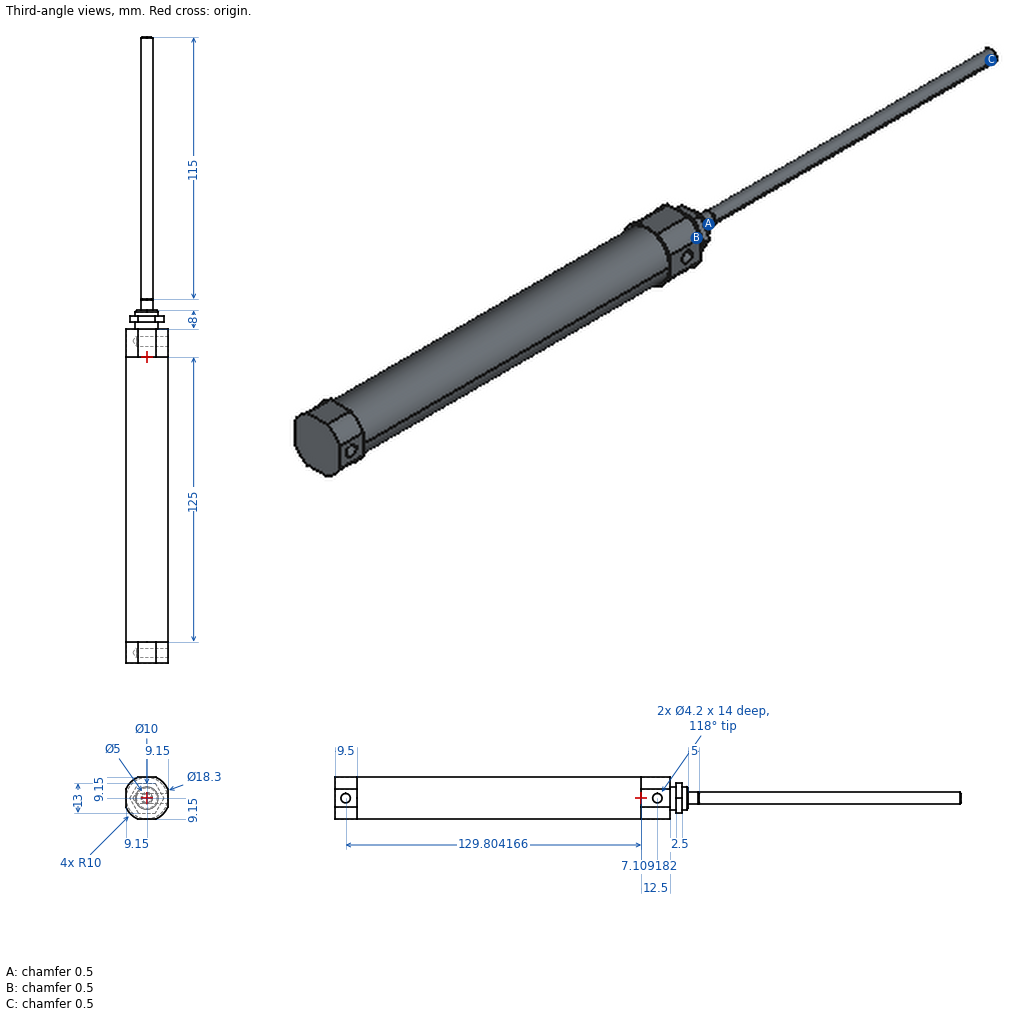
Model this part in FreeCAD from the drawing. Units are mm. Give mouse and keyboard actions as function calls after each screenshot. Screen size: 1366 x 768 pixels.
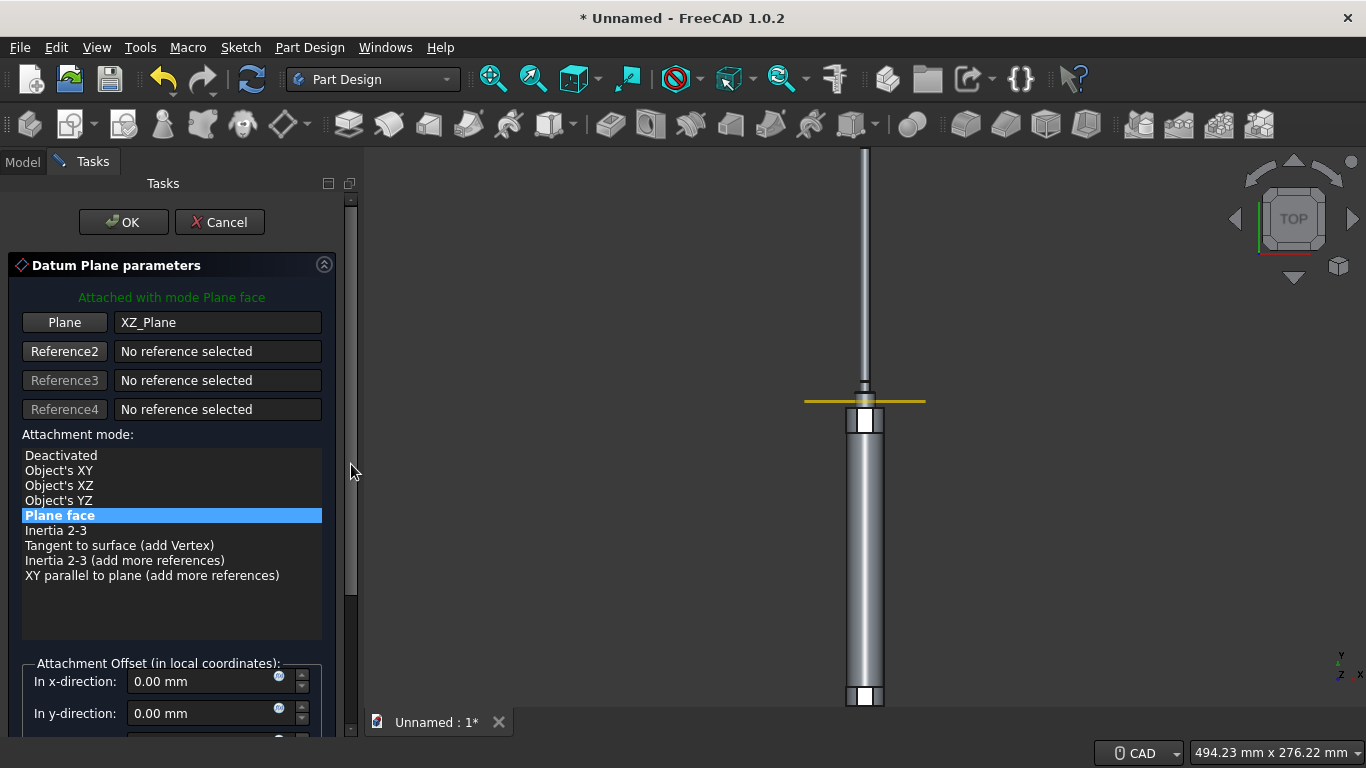
click(124, 222)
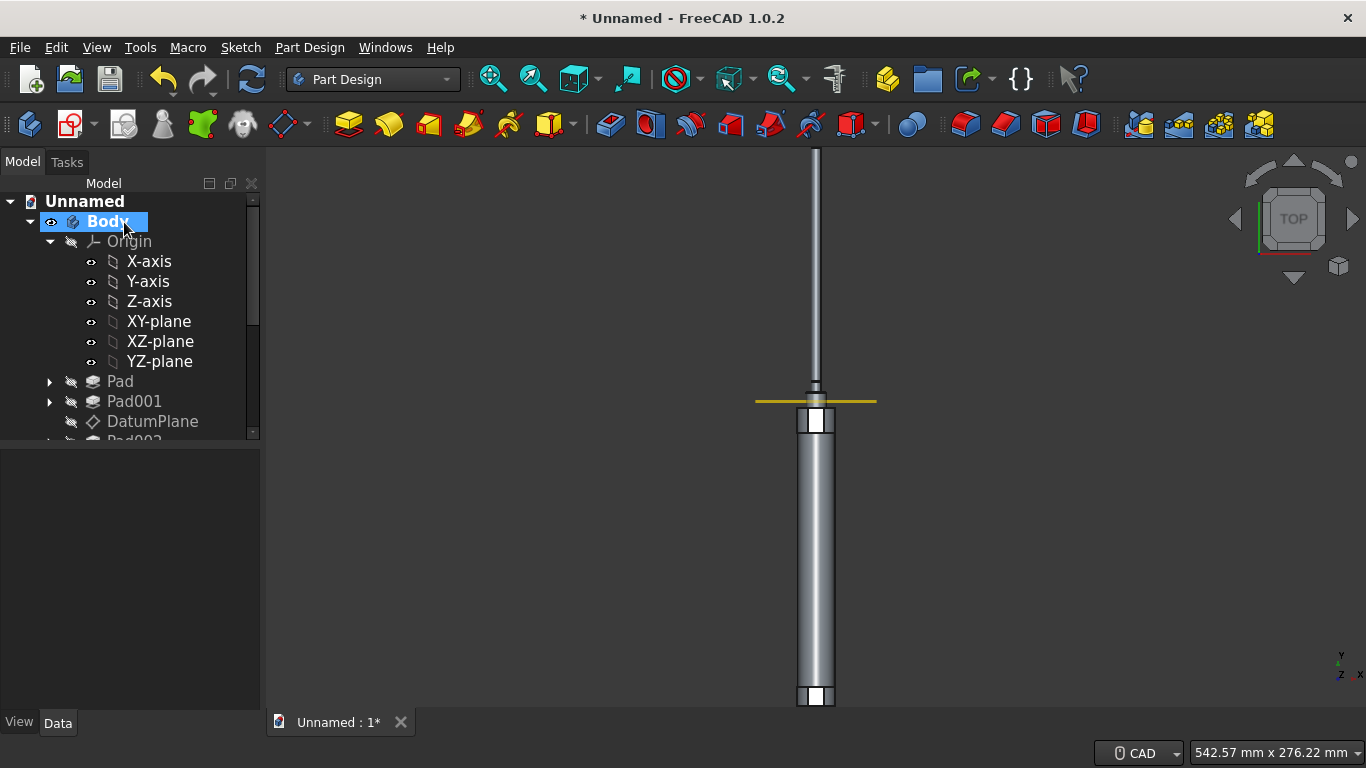
scroll(100, 317, down, 3)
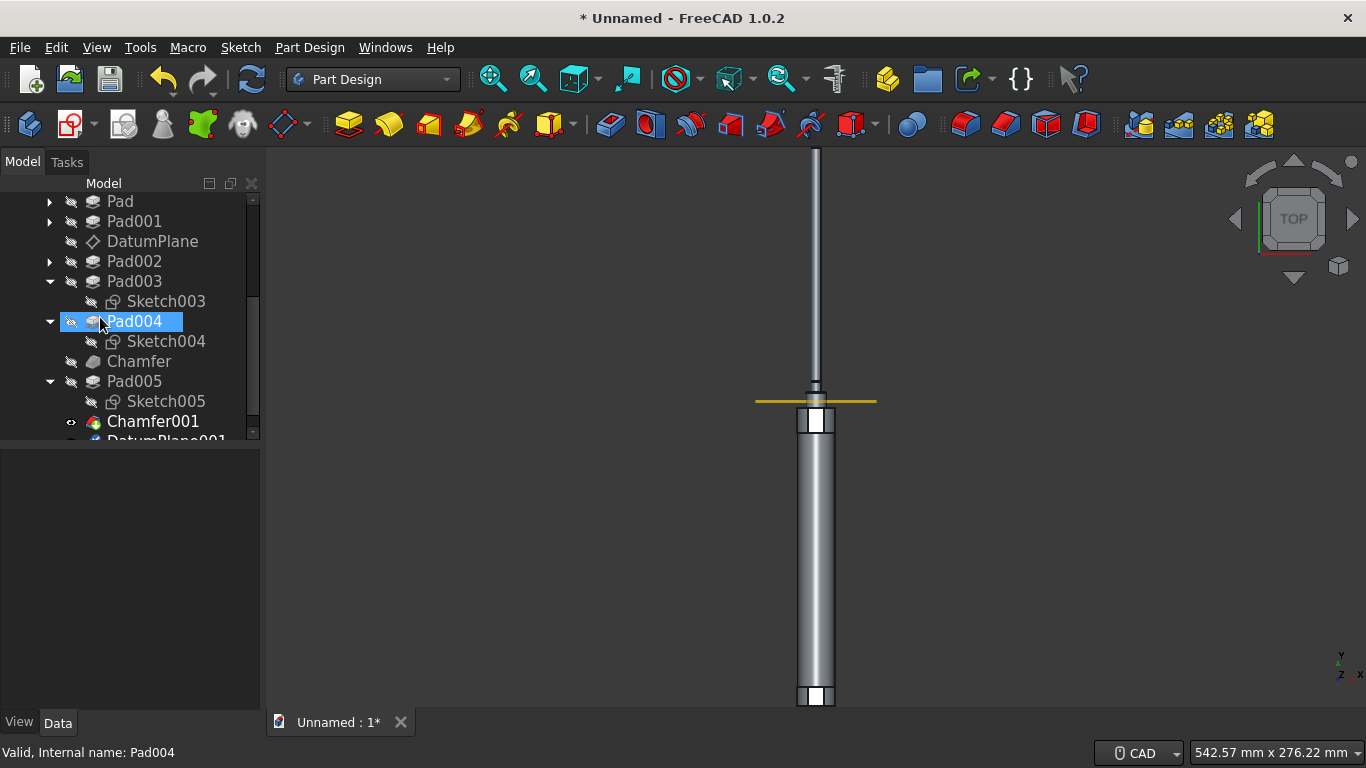
scroll(140, 317, up, 15)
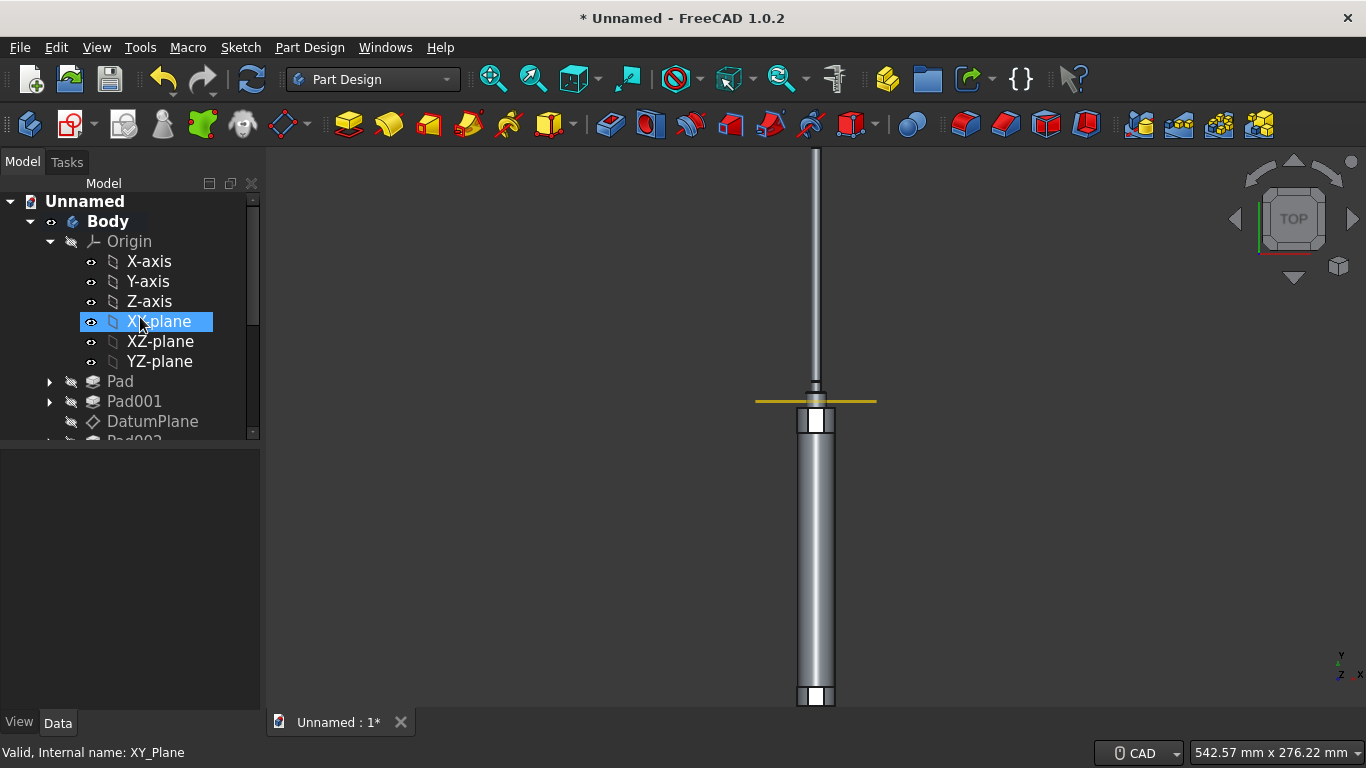
scroll(100, 317, down, 6)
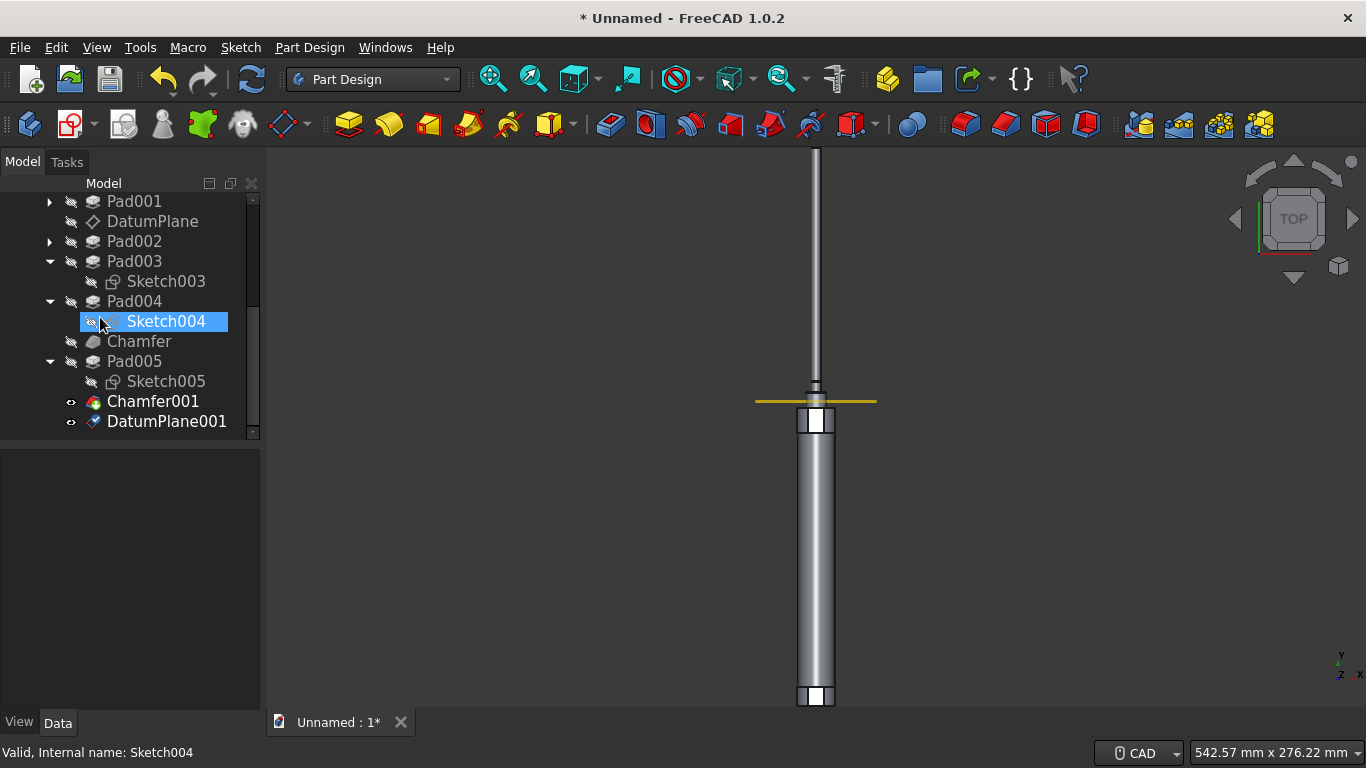
click(116, 422)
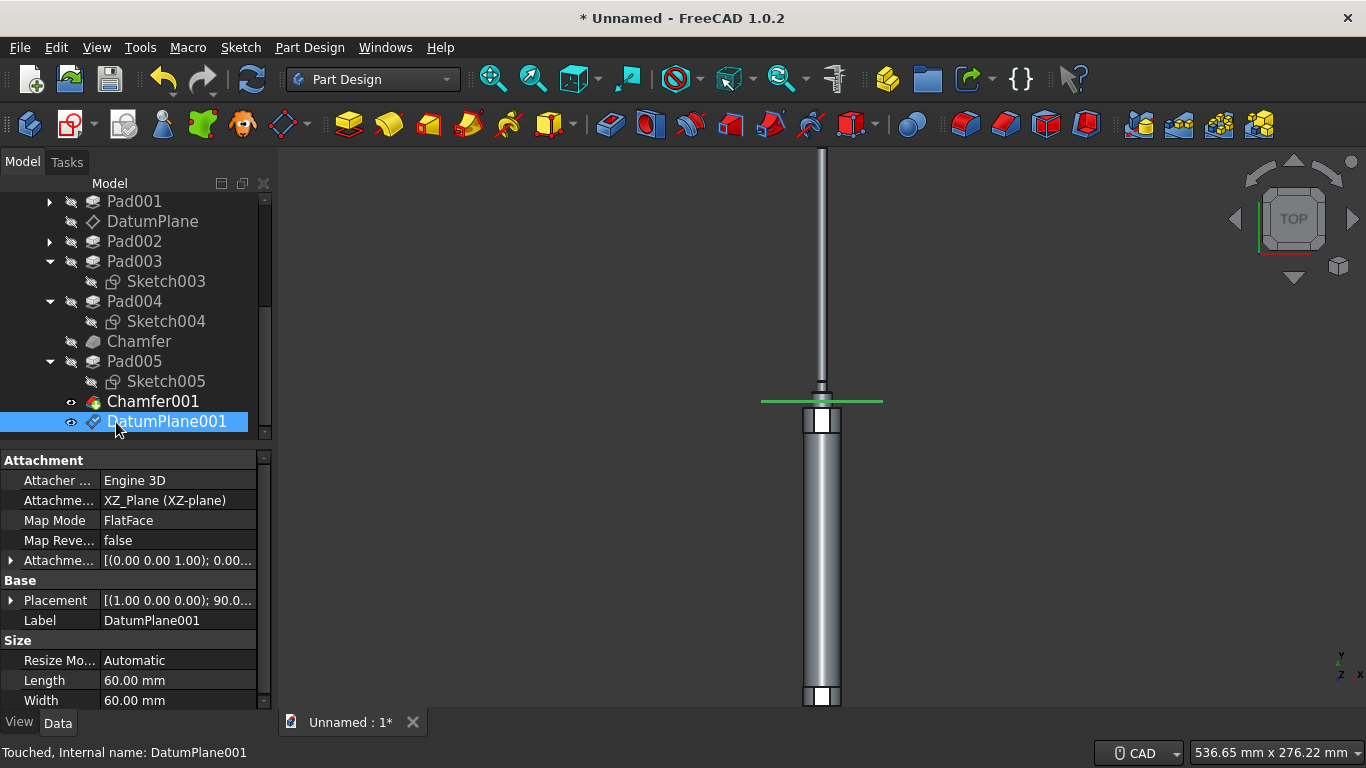
click(70, 124)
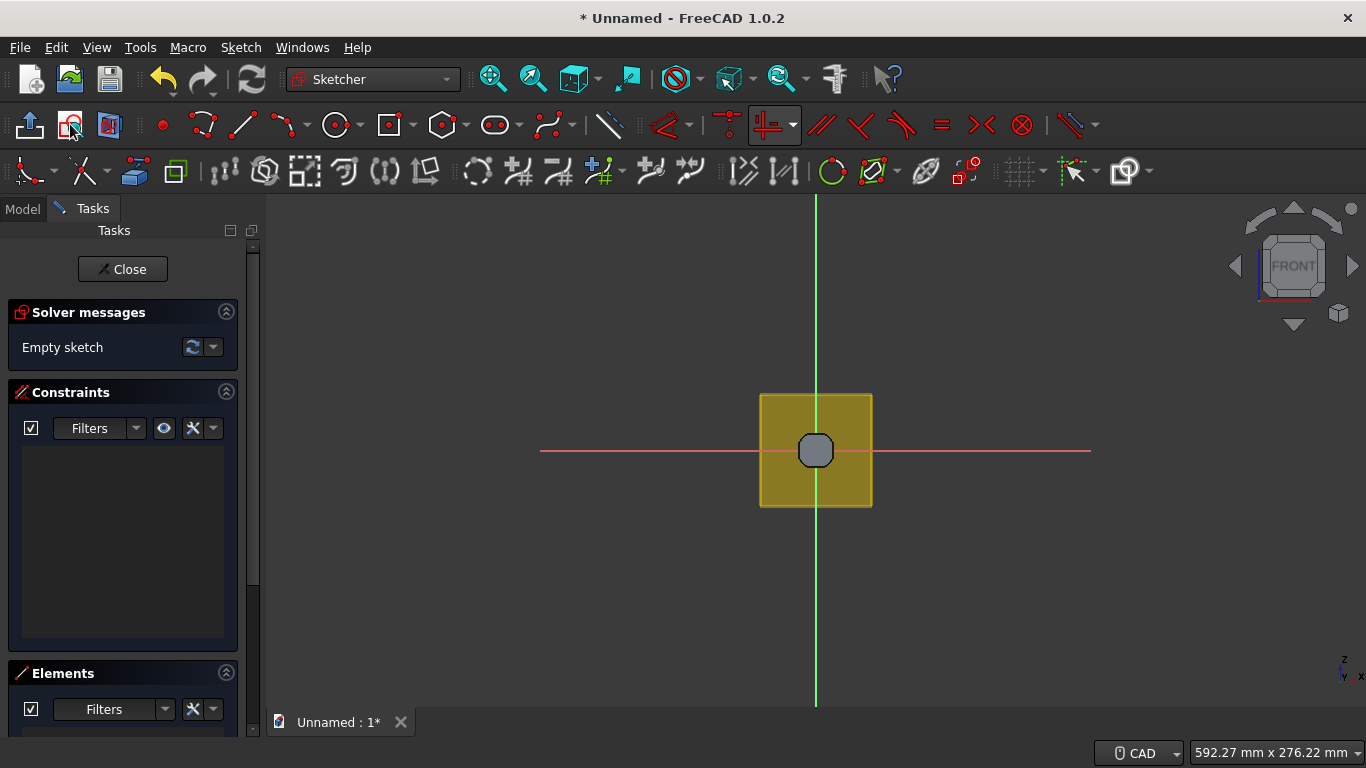
key(q)
key(s)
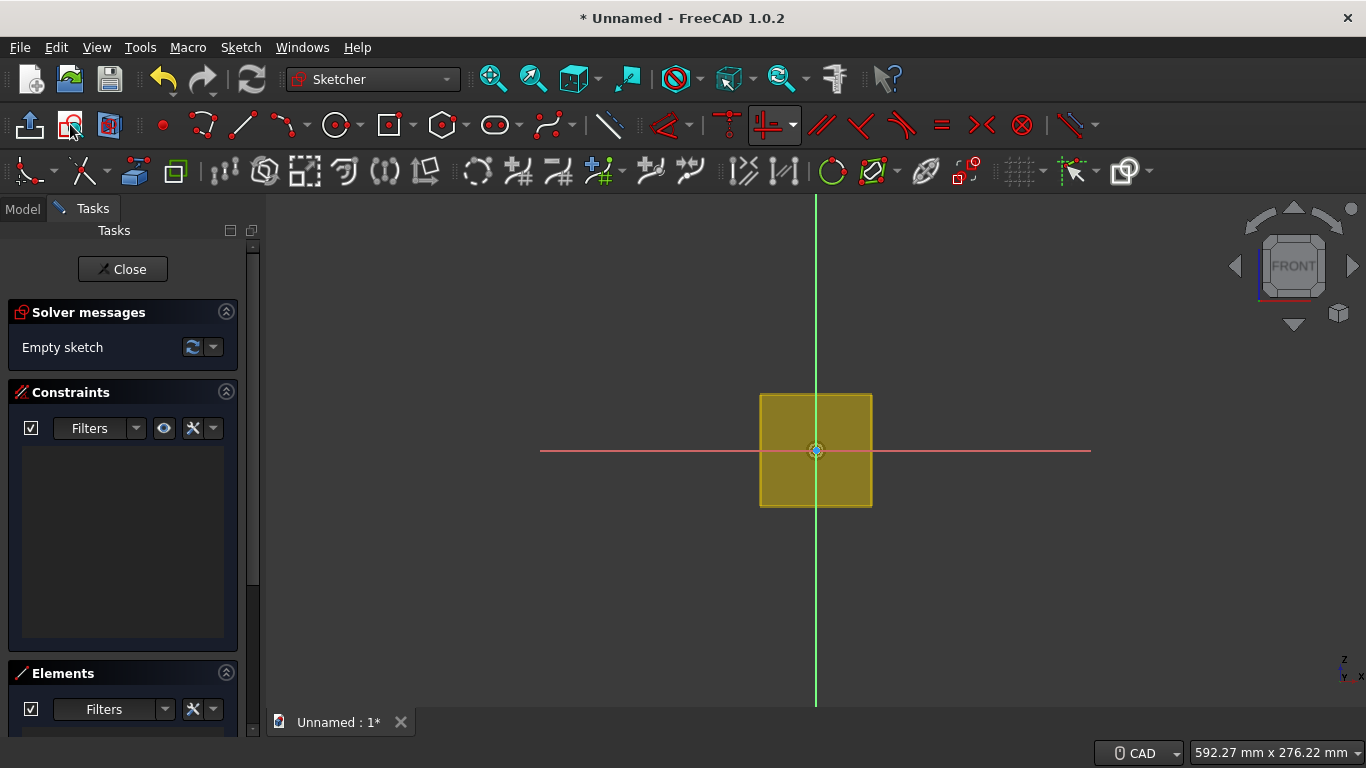
scroll(821, 450, up, 13)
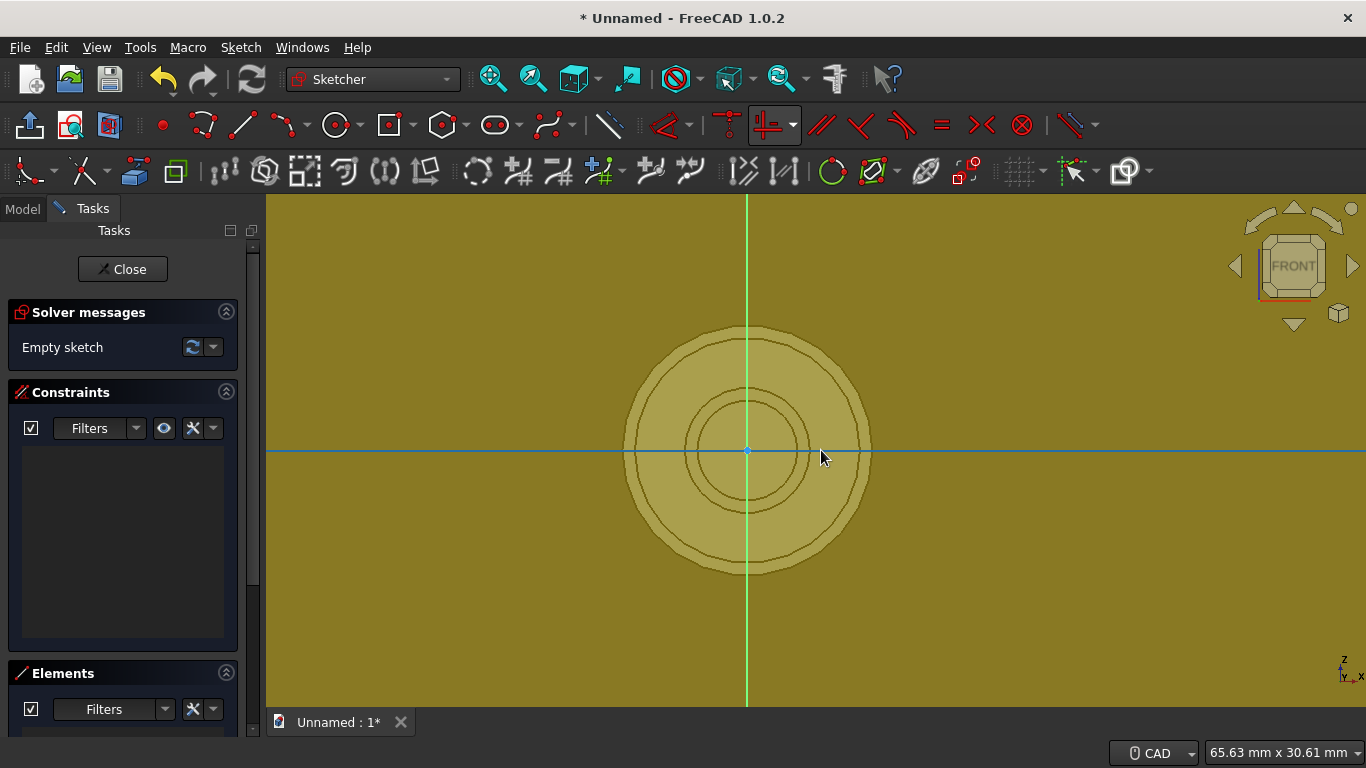
key(g)
key(p)
key(6)